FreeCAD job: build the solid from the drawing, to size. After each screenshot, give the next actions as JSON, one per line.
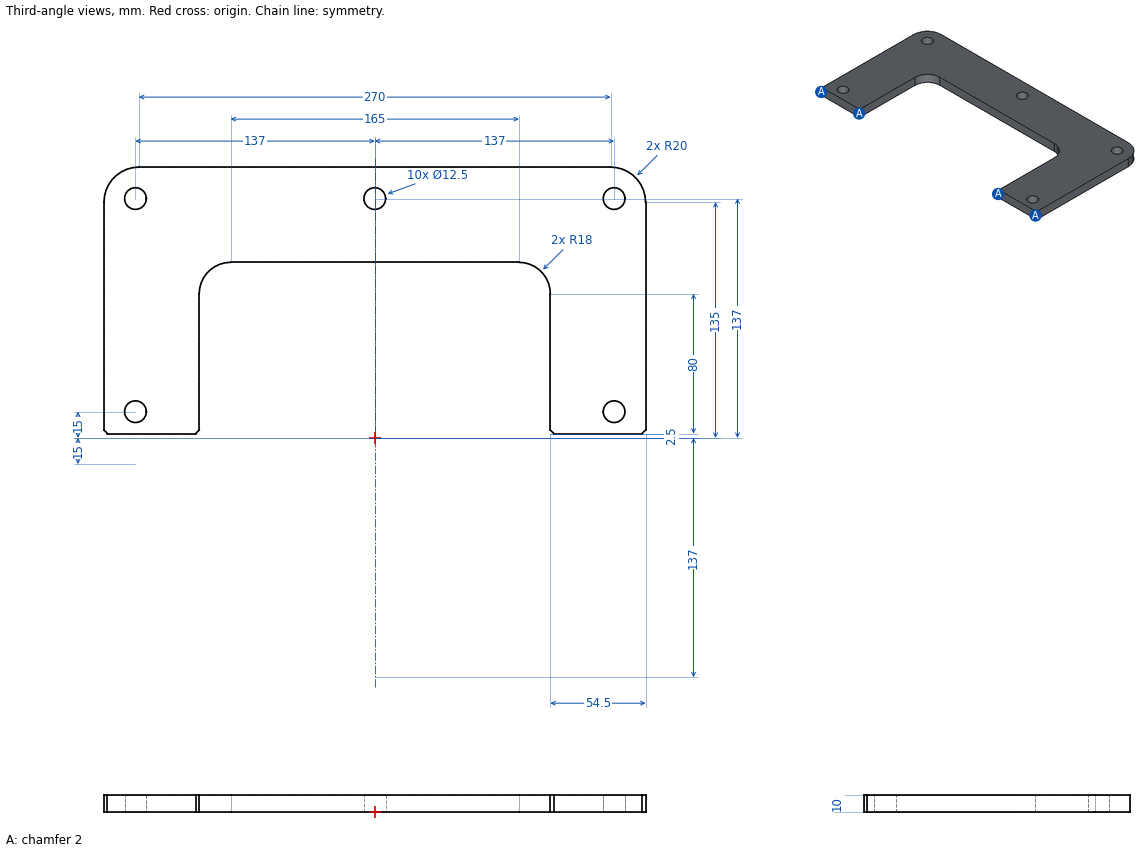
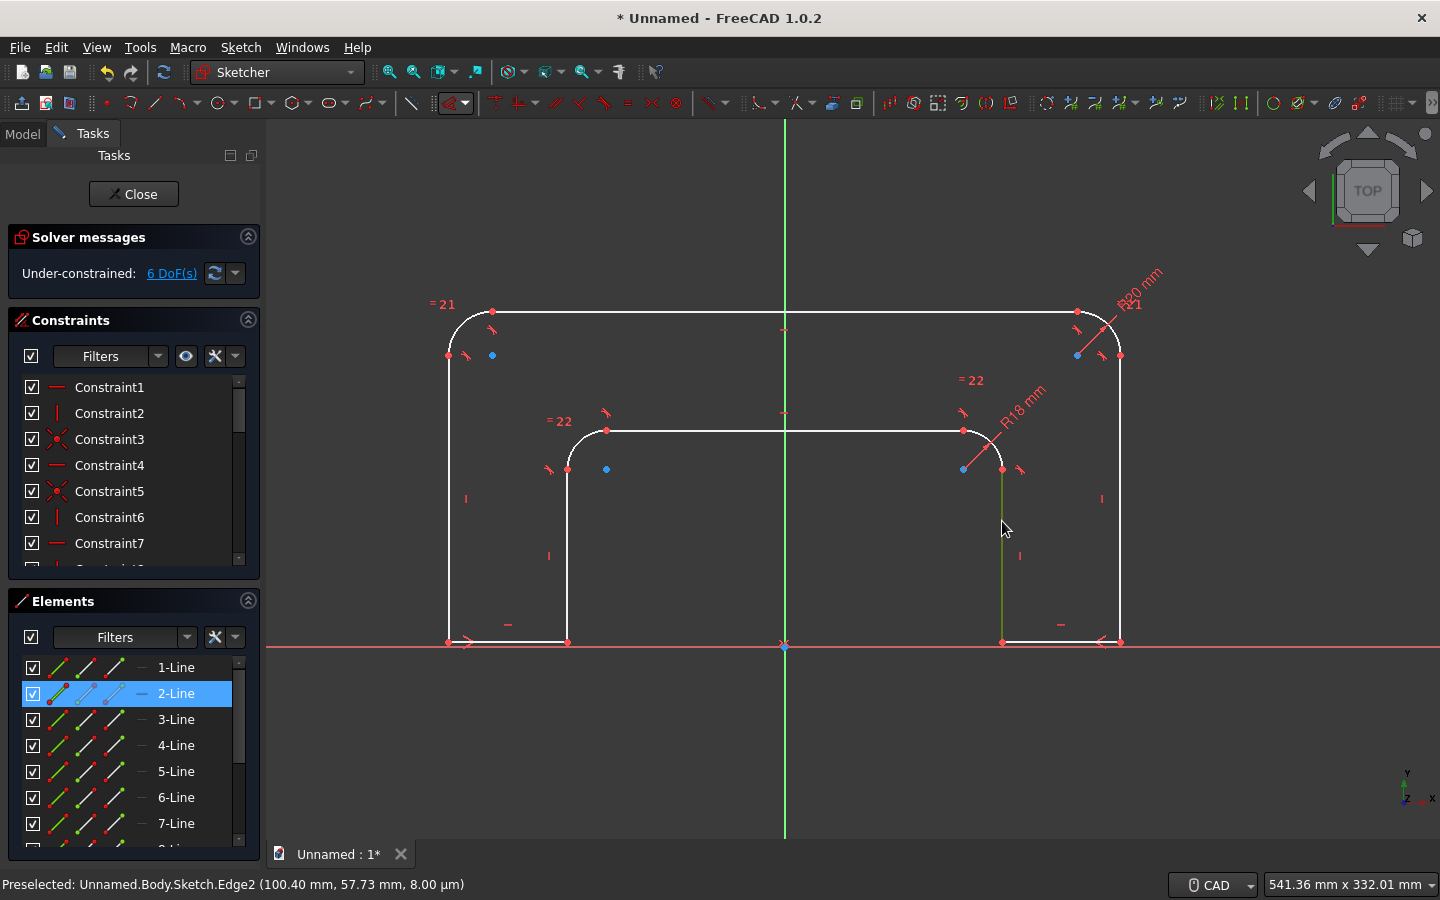
{"action": "key", "text": "i"}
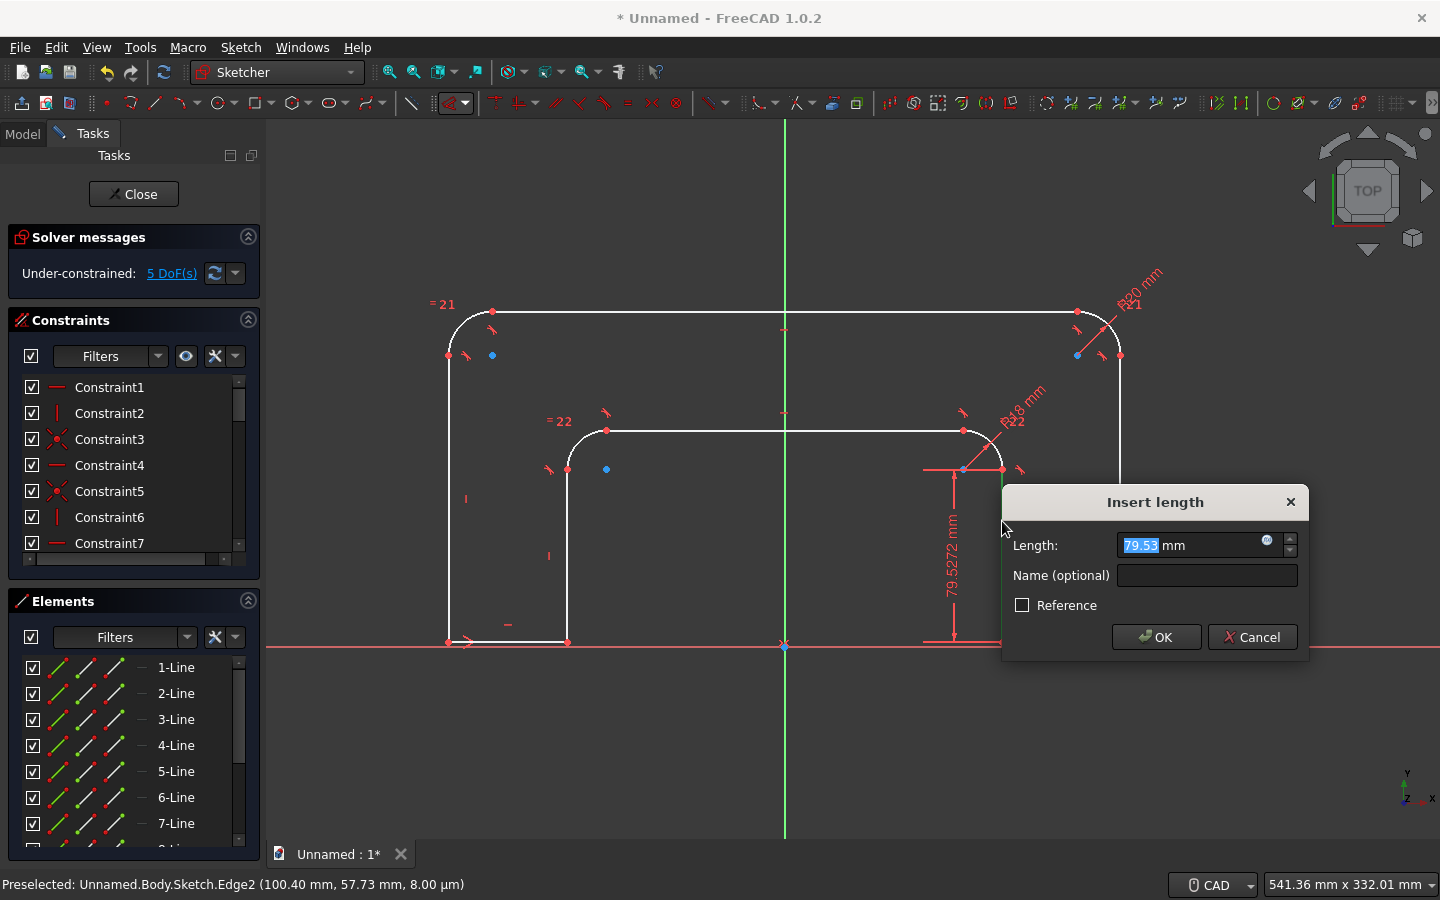
{"action": "type", "text": "80"}
{"action": "key", "text": "Return"}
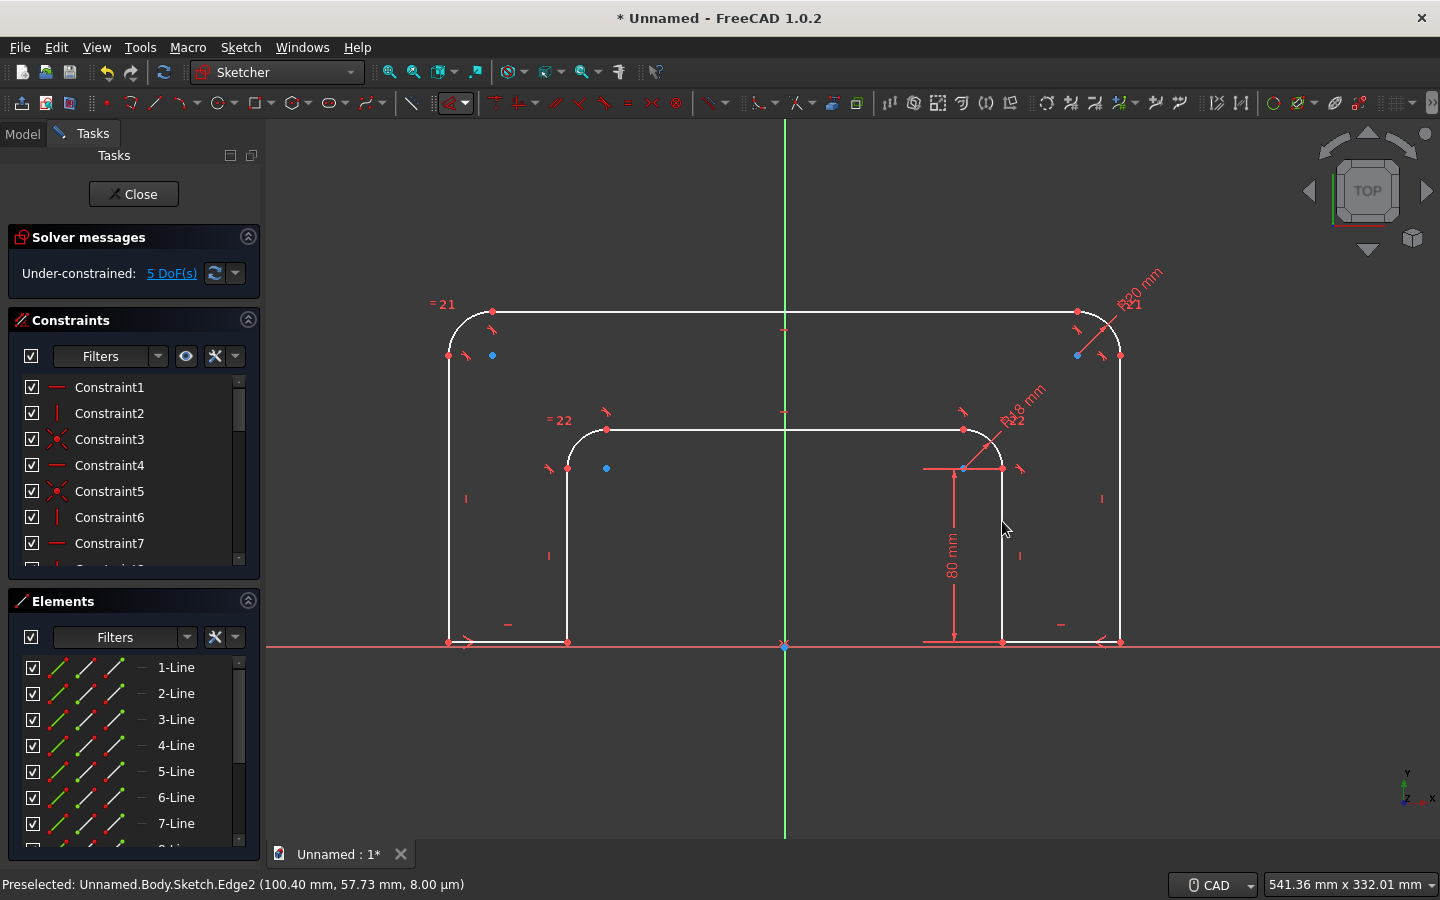
{"action": "left_click", "coordinate": [714, 430]}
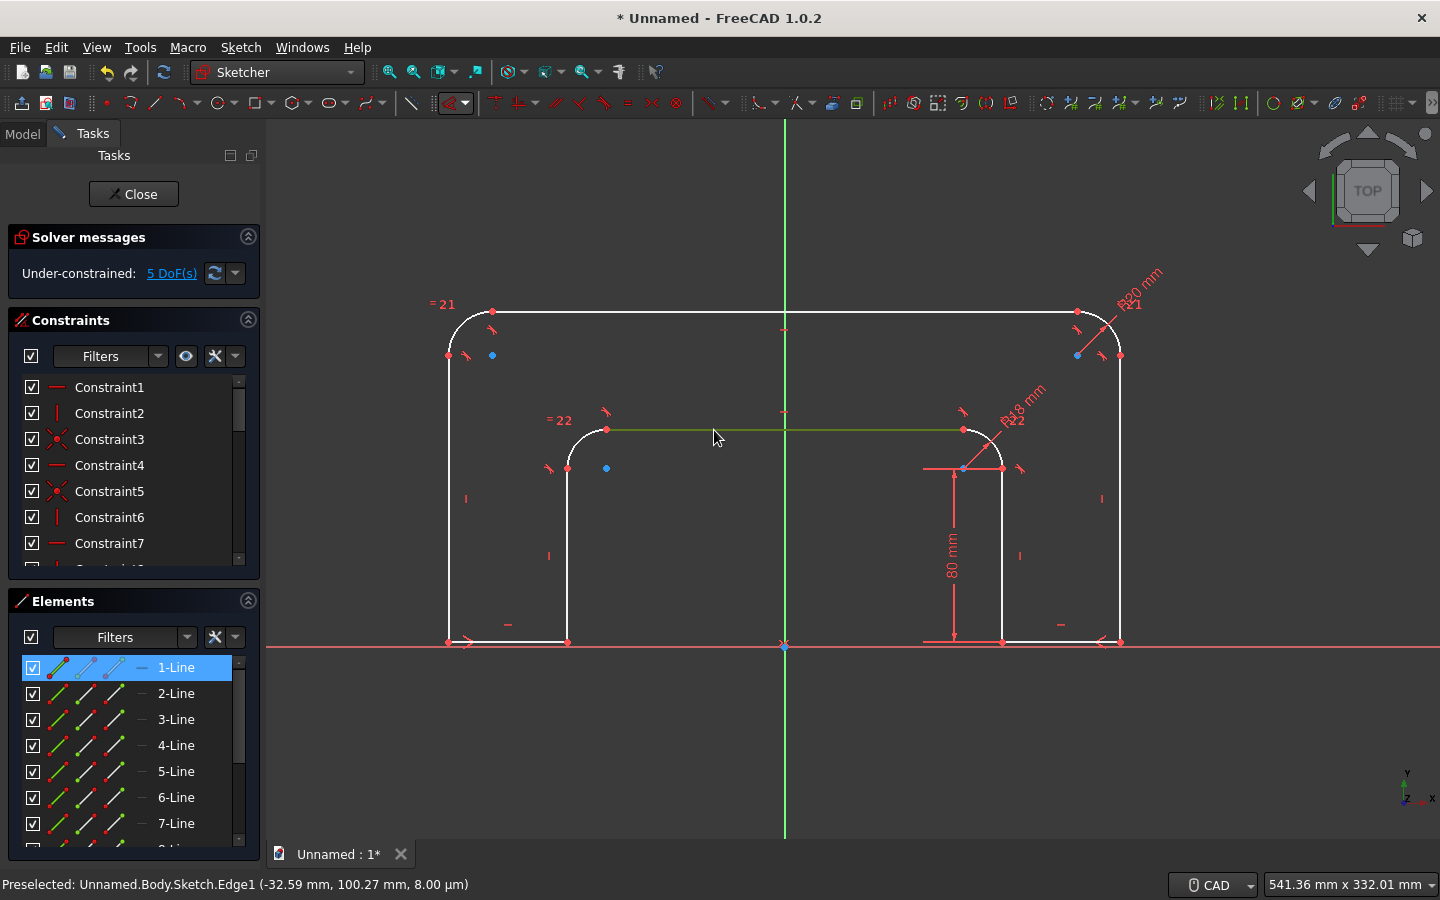
{"action": "key", "text": "l"}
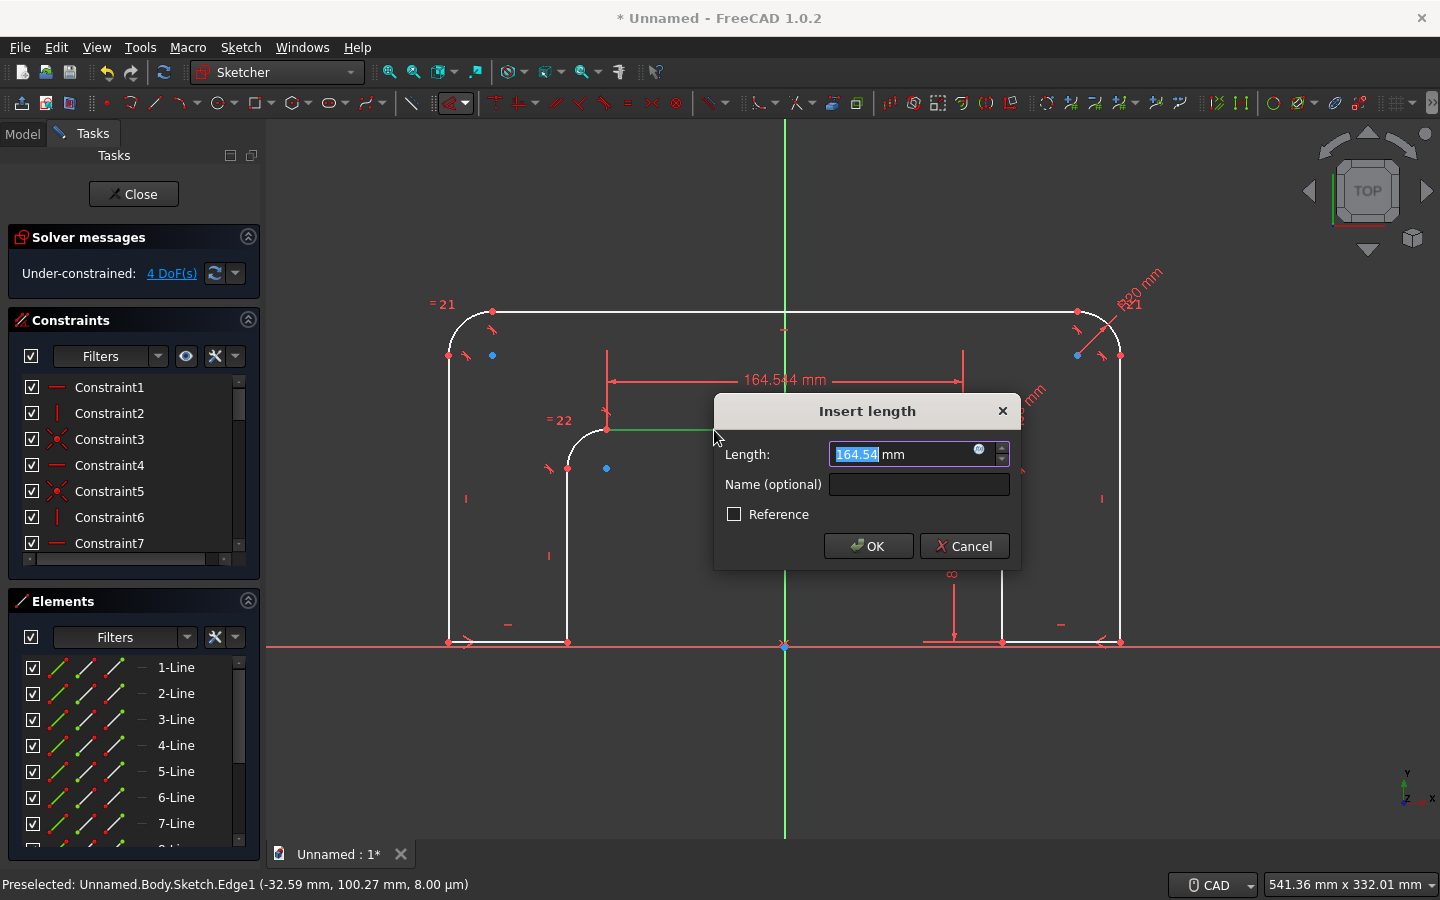
{"action": "type", "text": "165"}
{"action": "key", "text": "Return"}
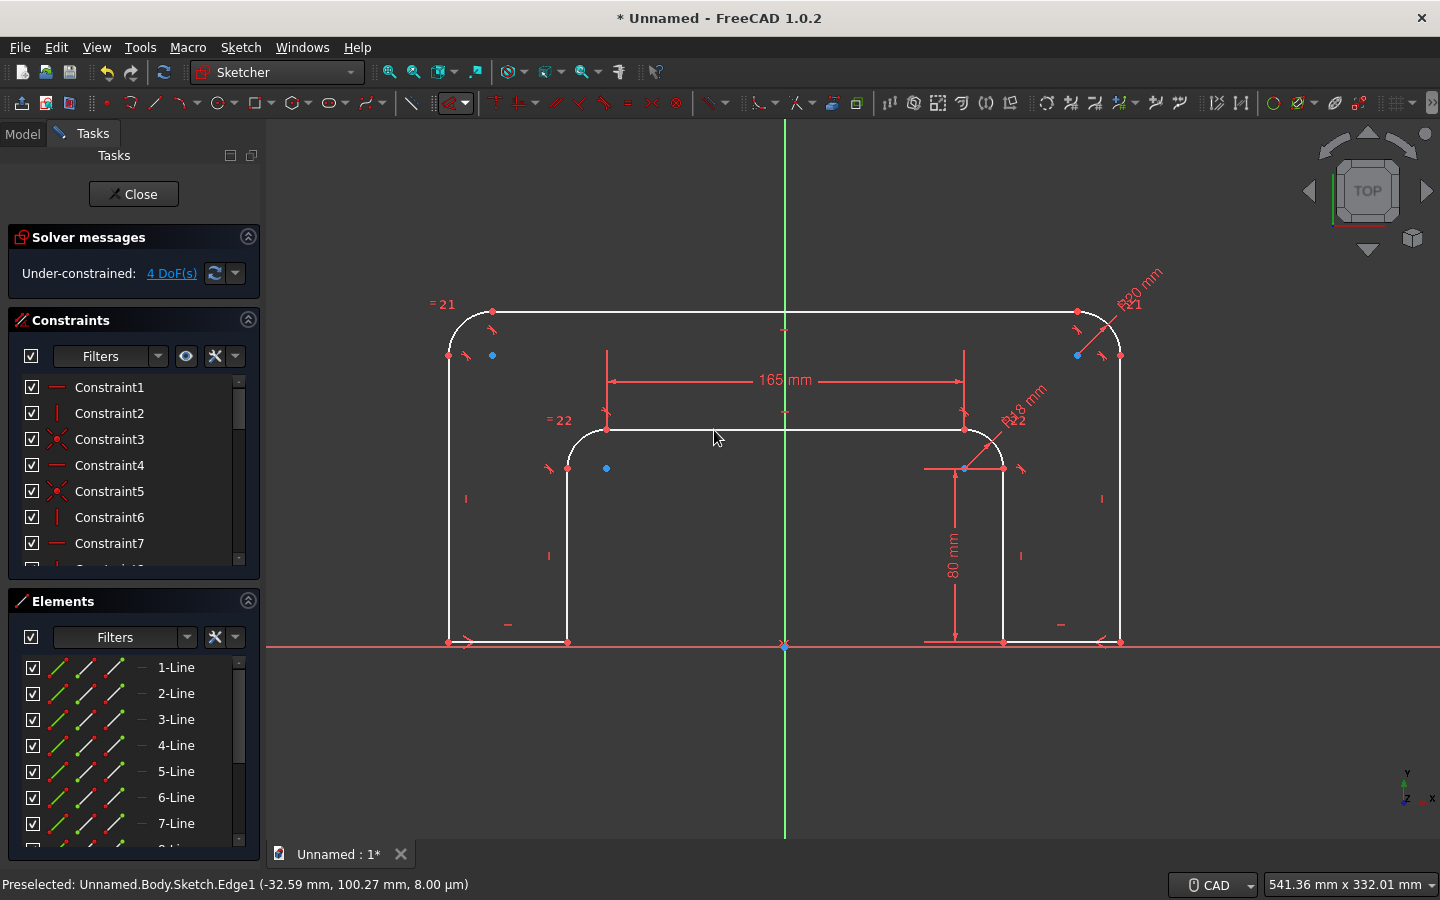
{"action": "left_click", "coordinate": [902, 312]}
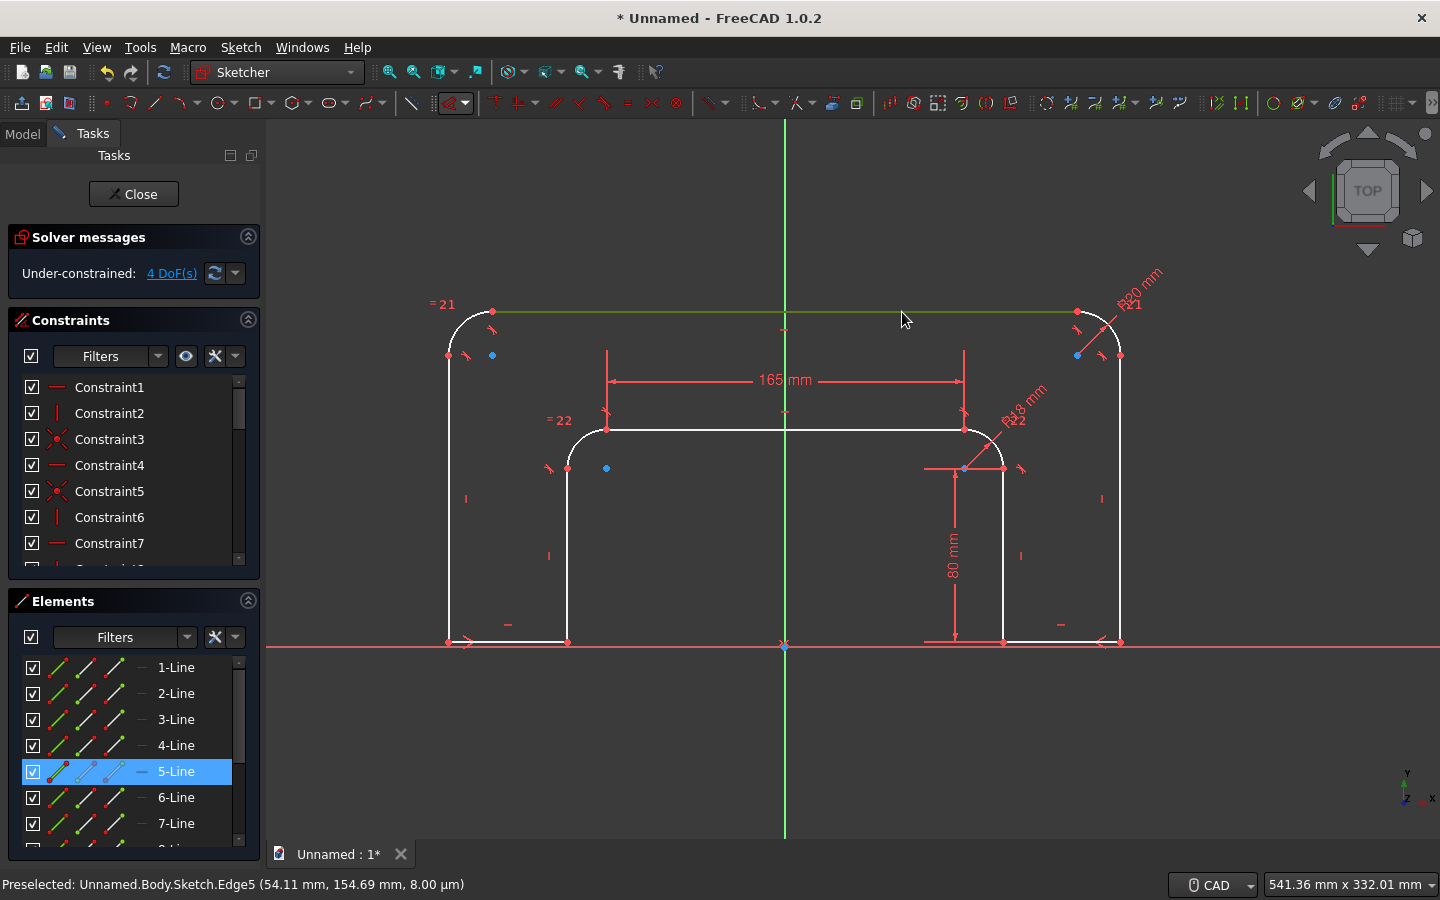
{"action": "left_click", "coordinate": [468, 104]}